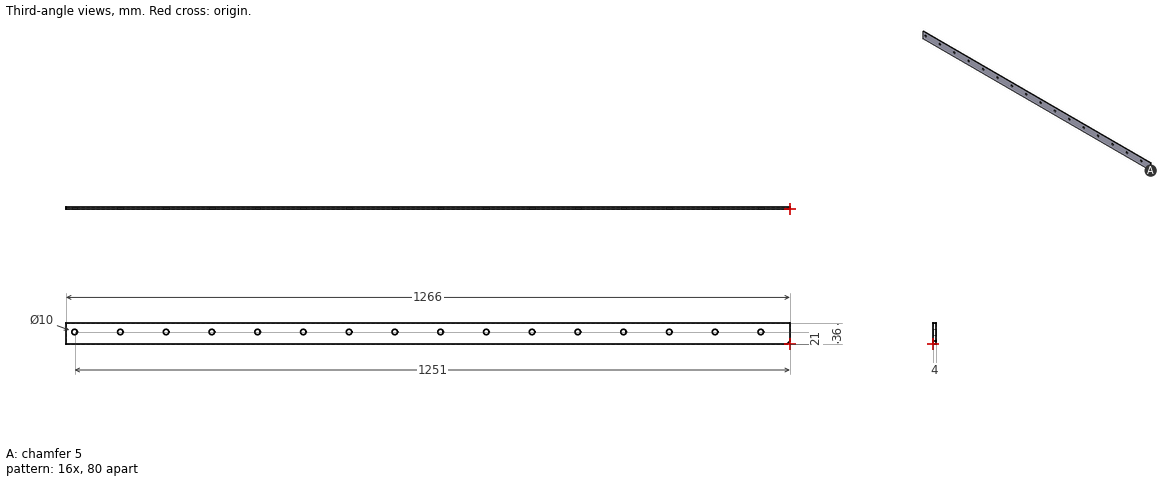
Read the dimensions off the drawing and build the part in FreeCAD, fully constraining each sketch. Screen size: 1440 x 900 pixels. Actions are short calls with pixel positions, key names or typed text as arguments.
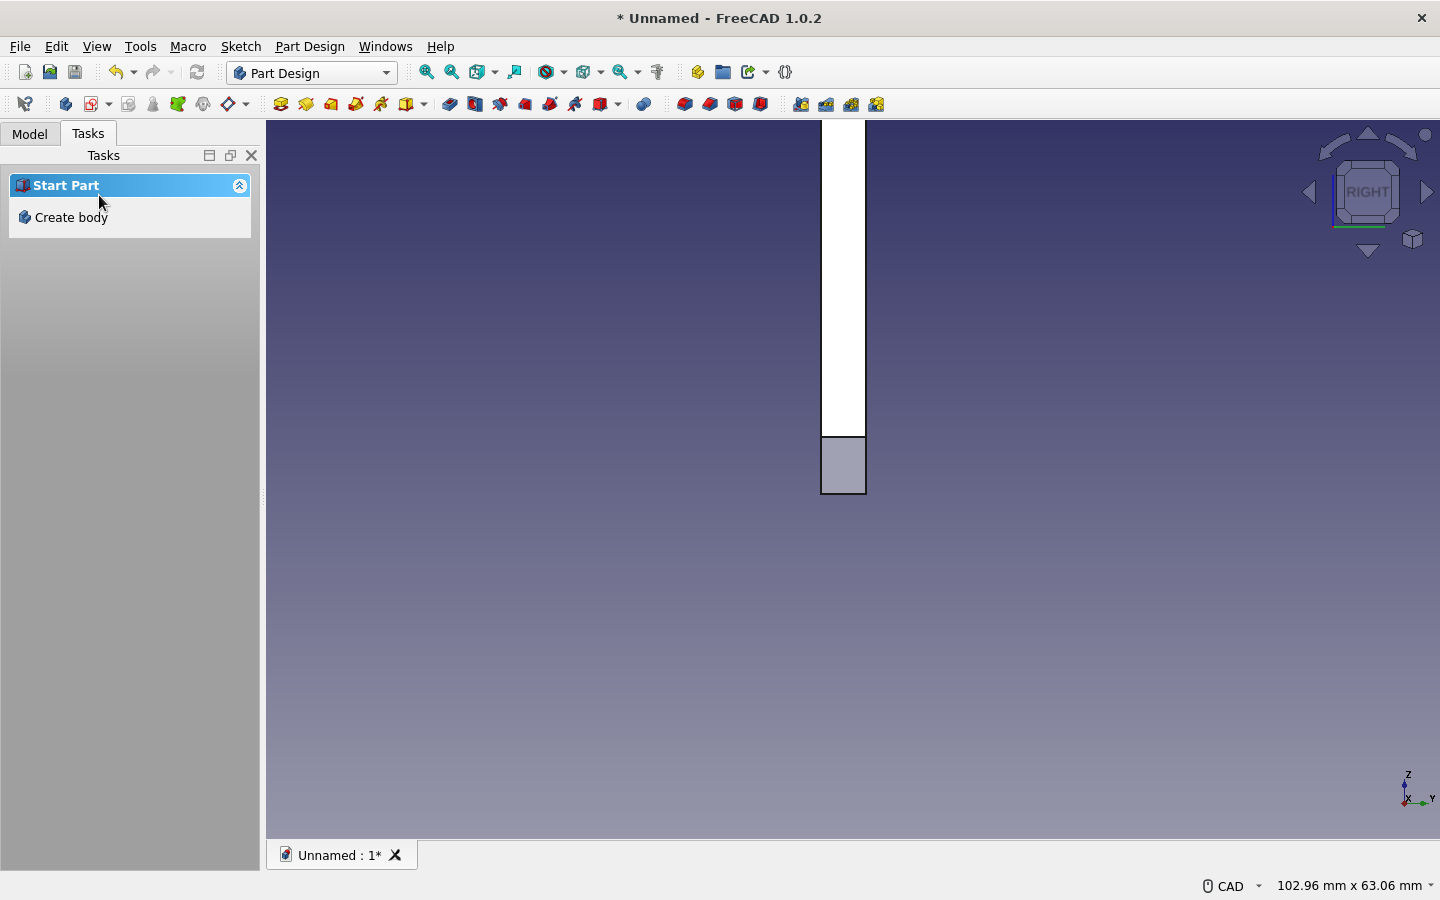
click(427, 72)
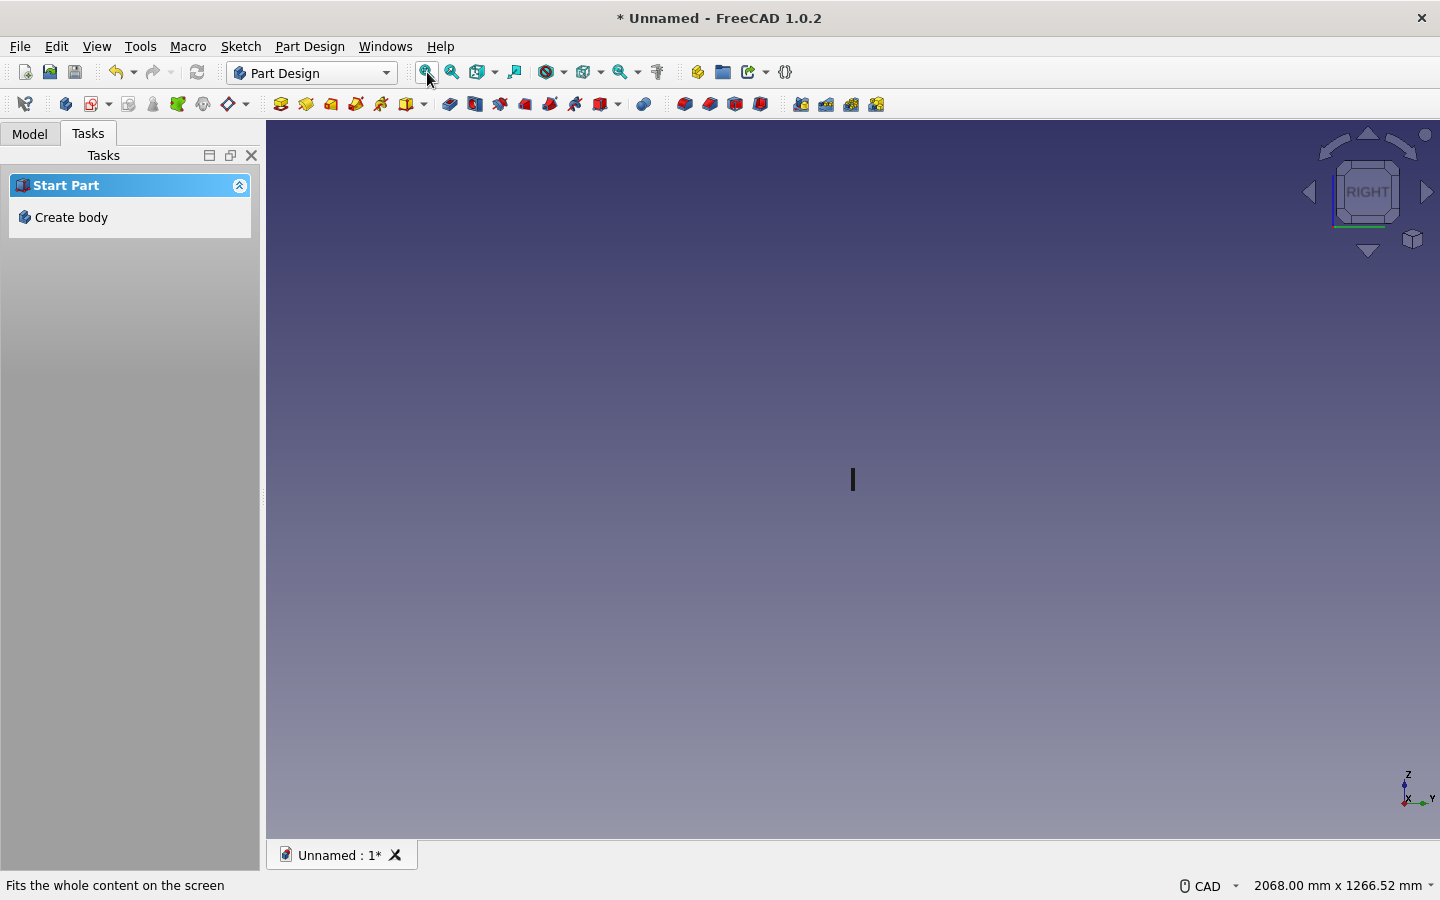
key(4)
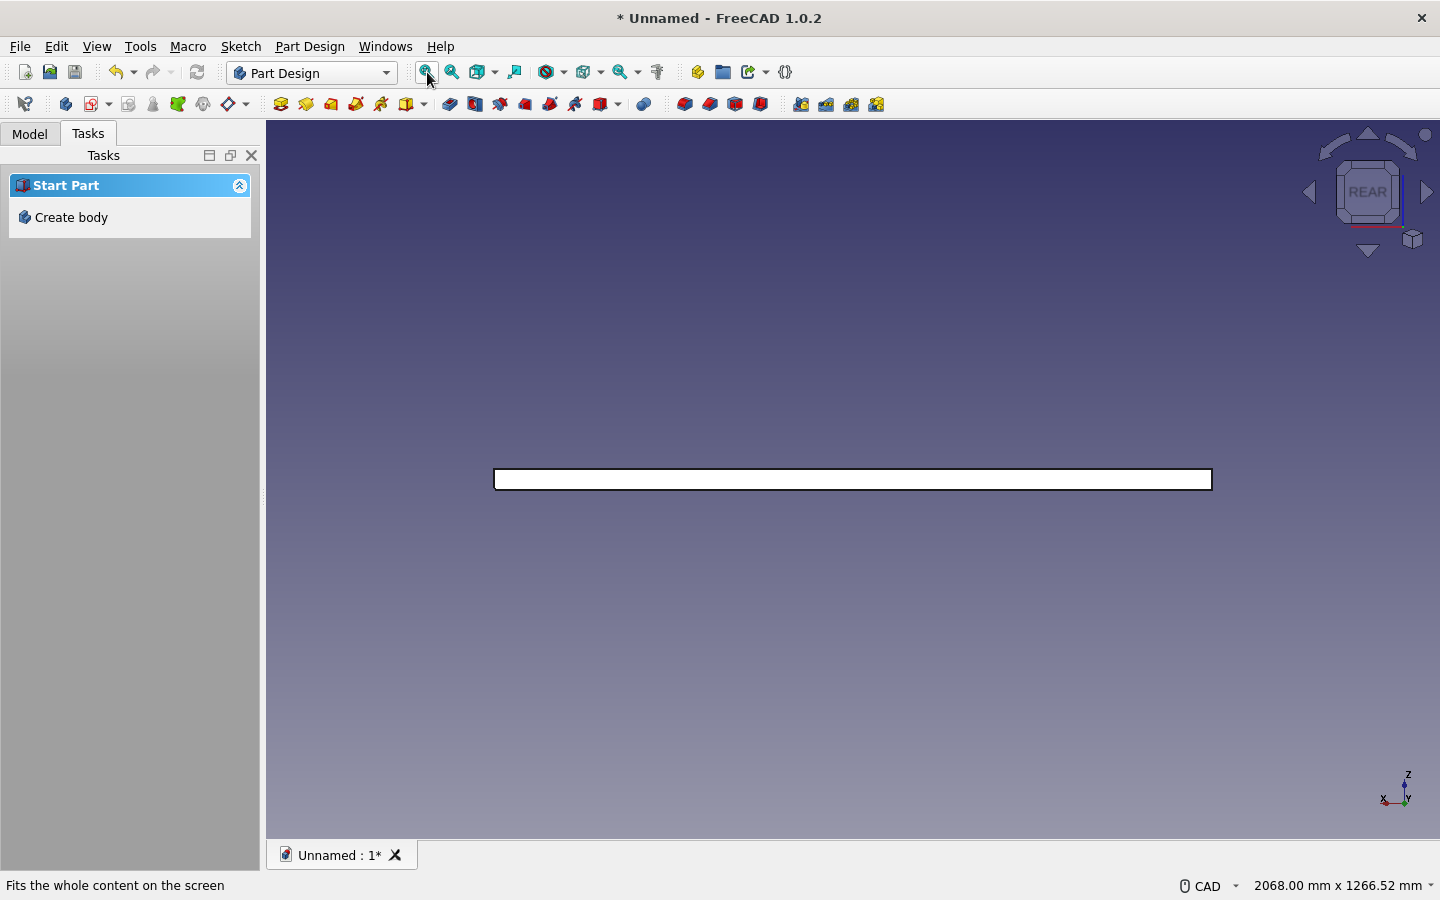
click(545, 479)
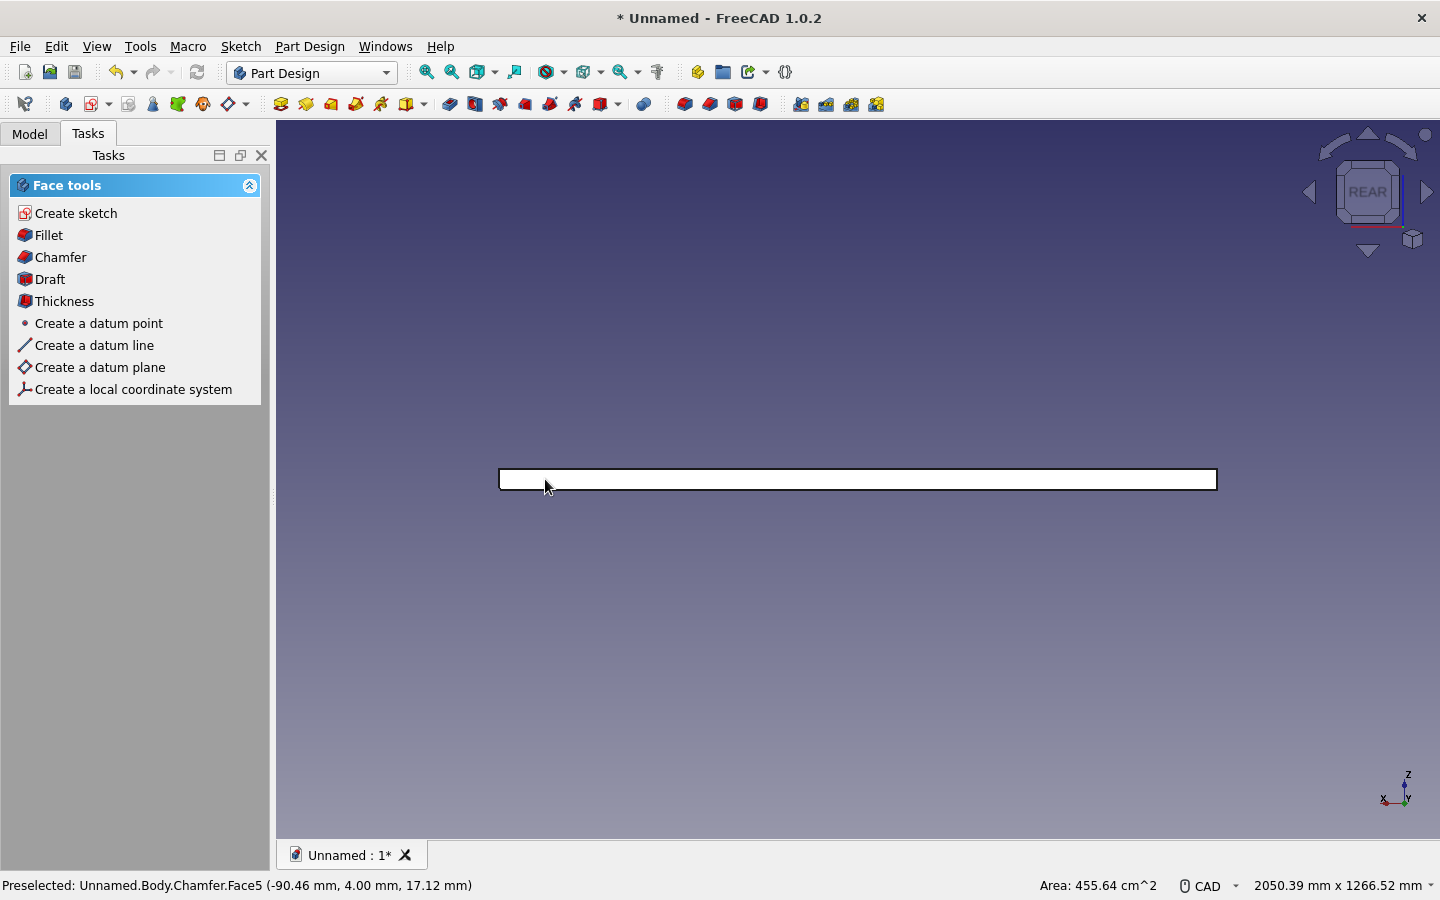
click(90, 104)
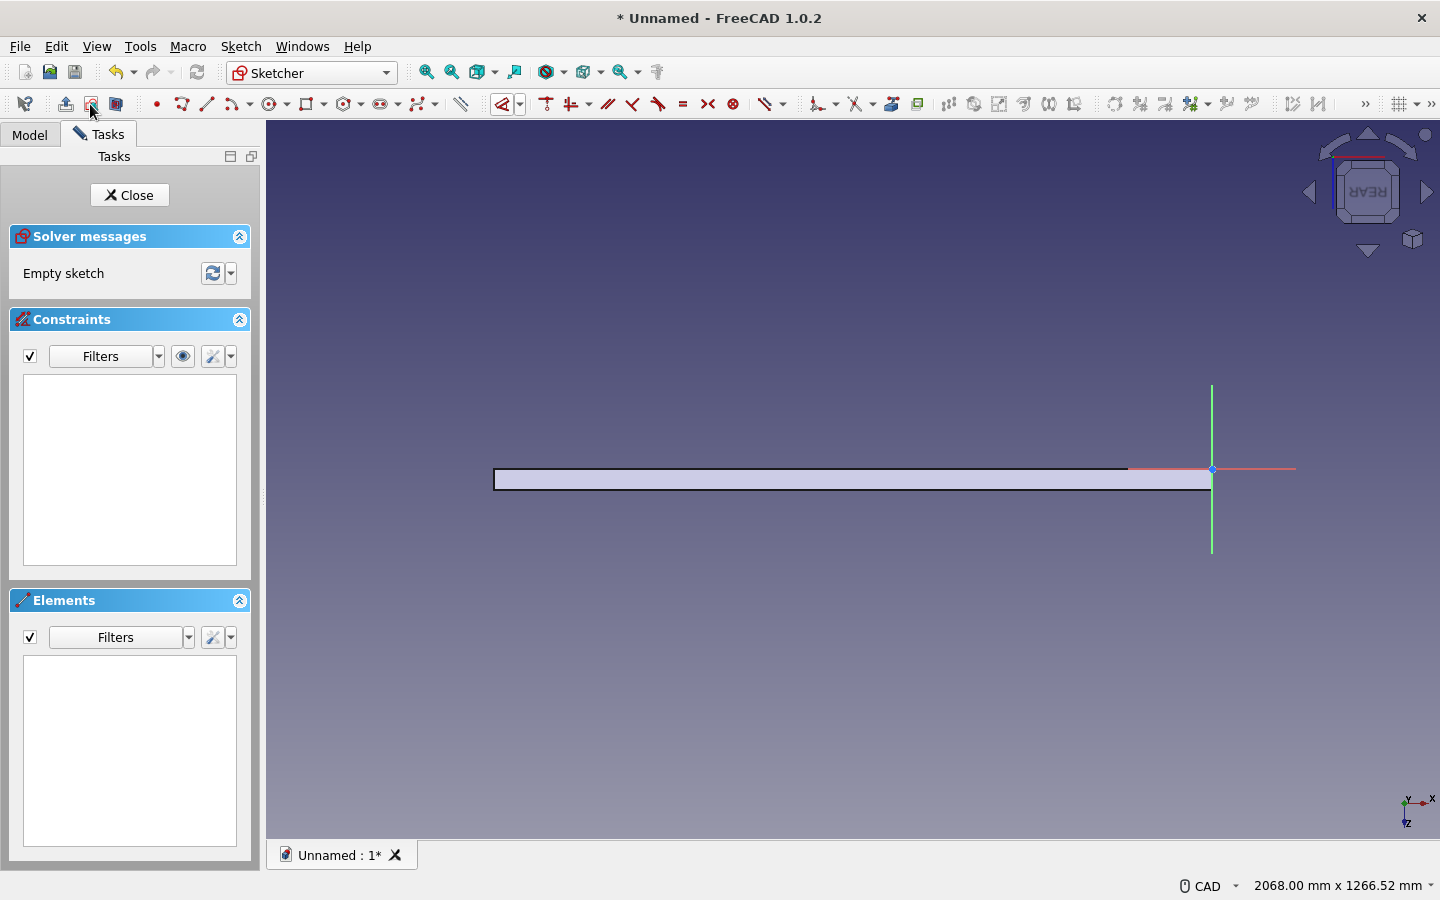
scroll(487, 481, up, 15)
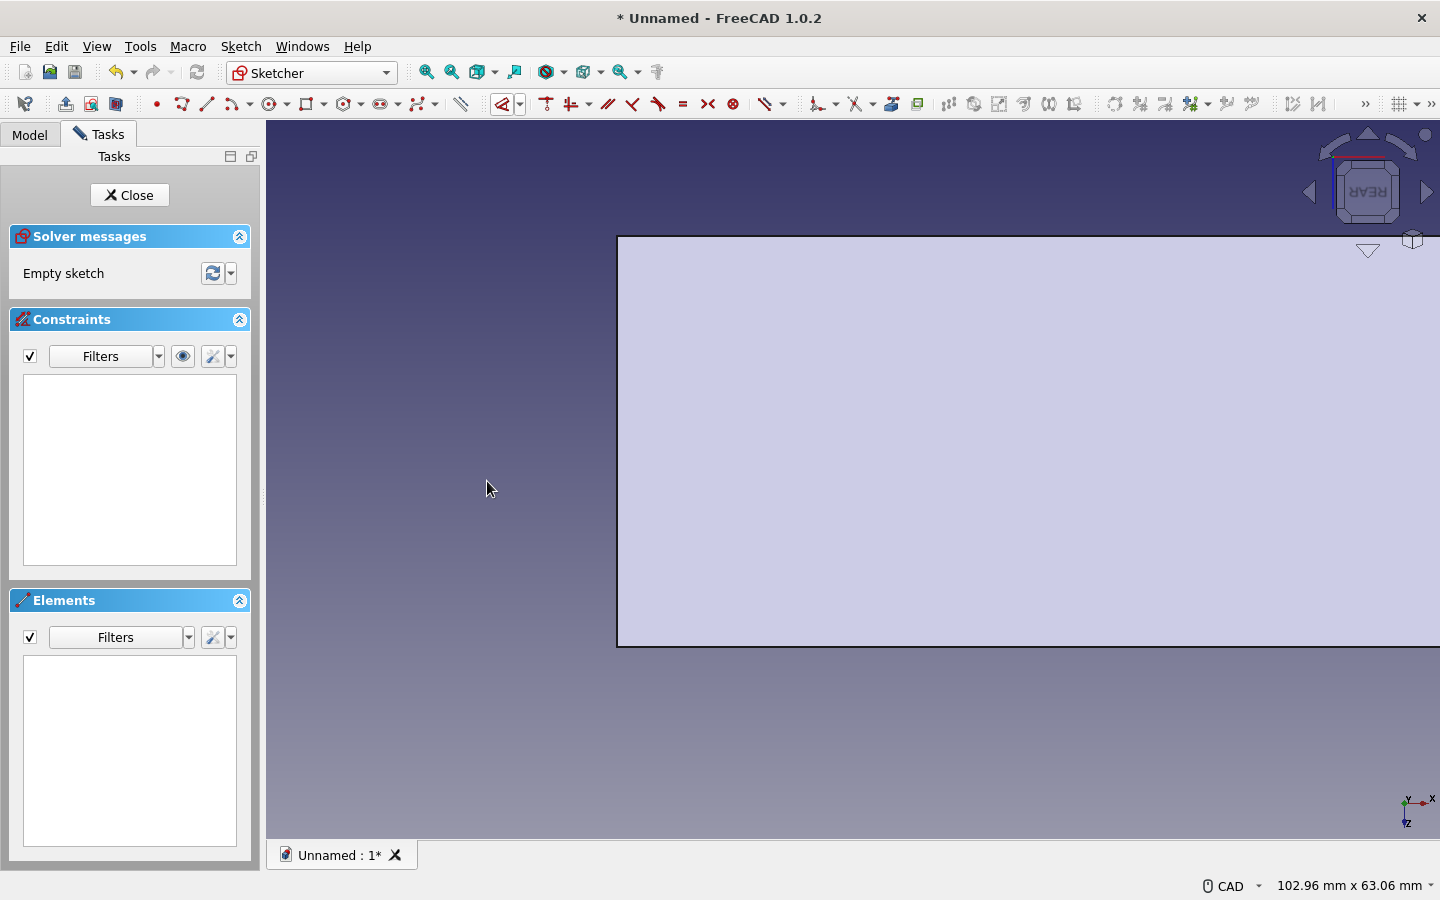
scroll(789, 474, up, 7)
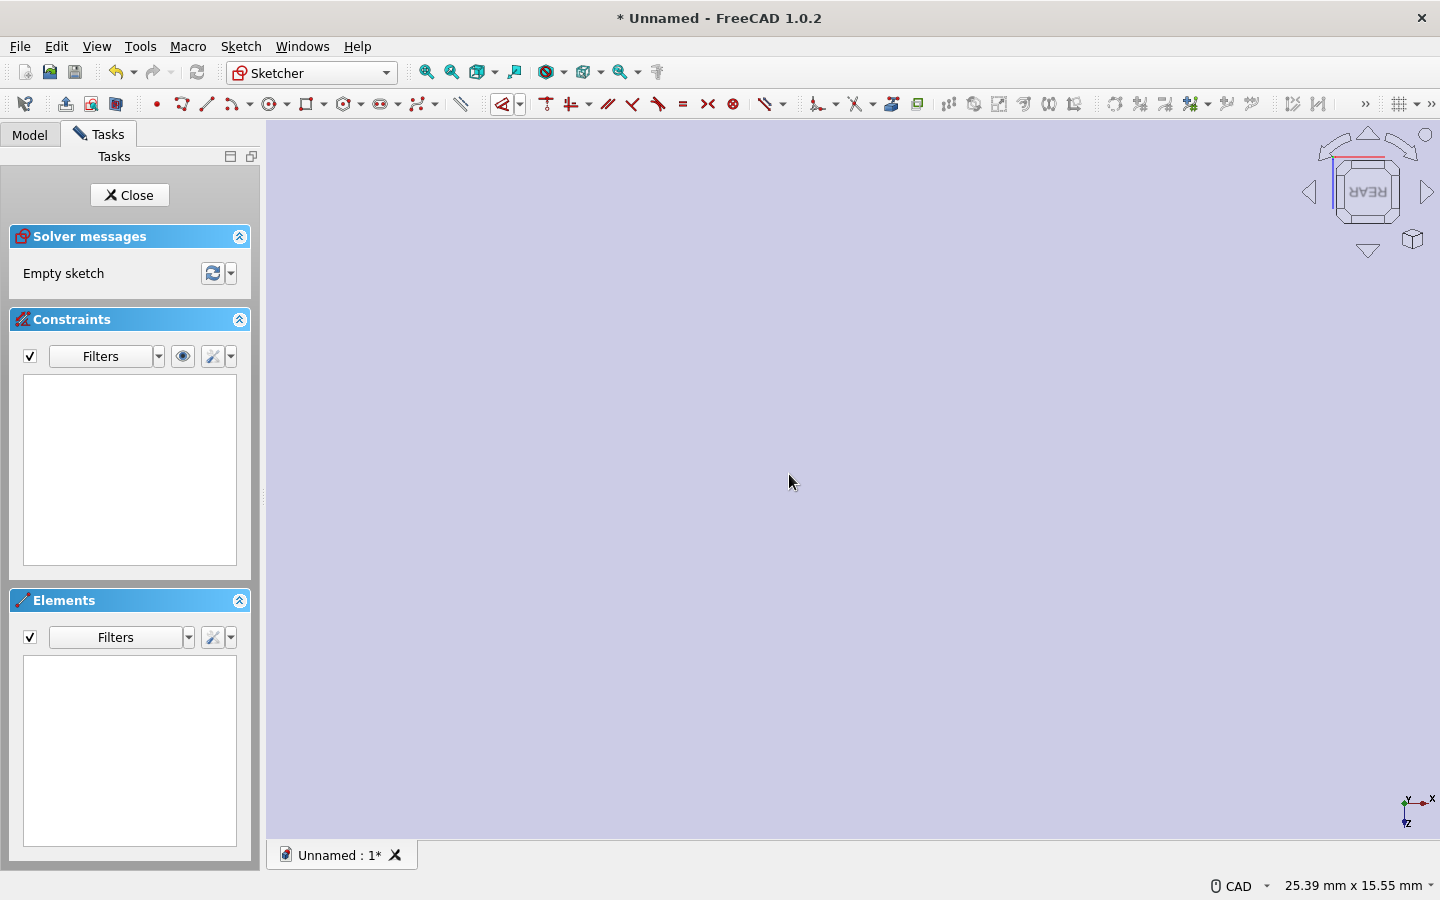
click(268, 104)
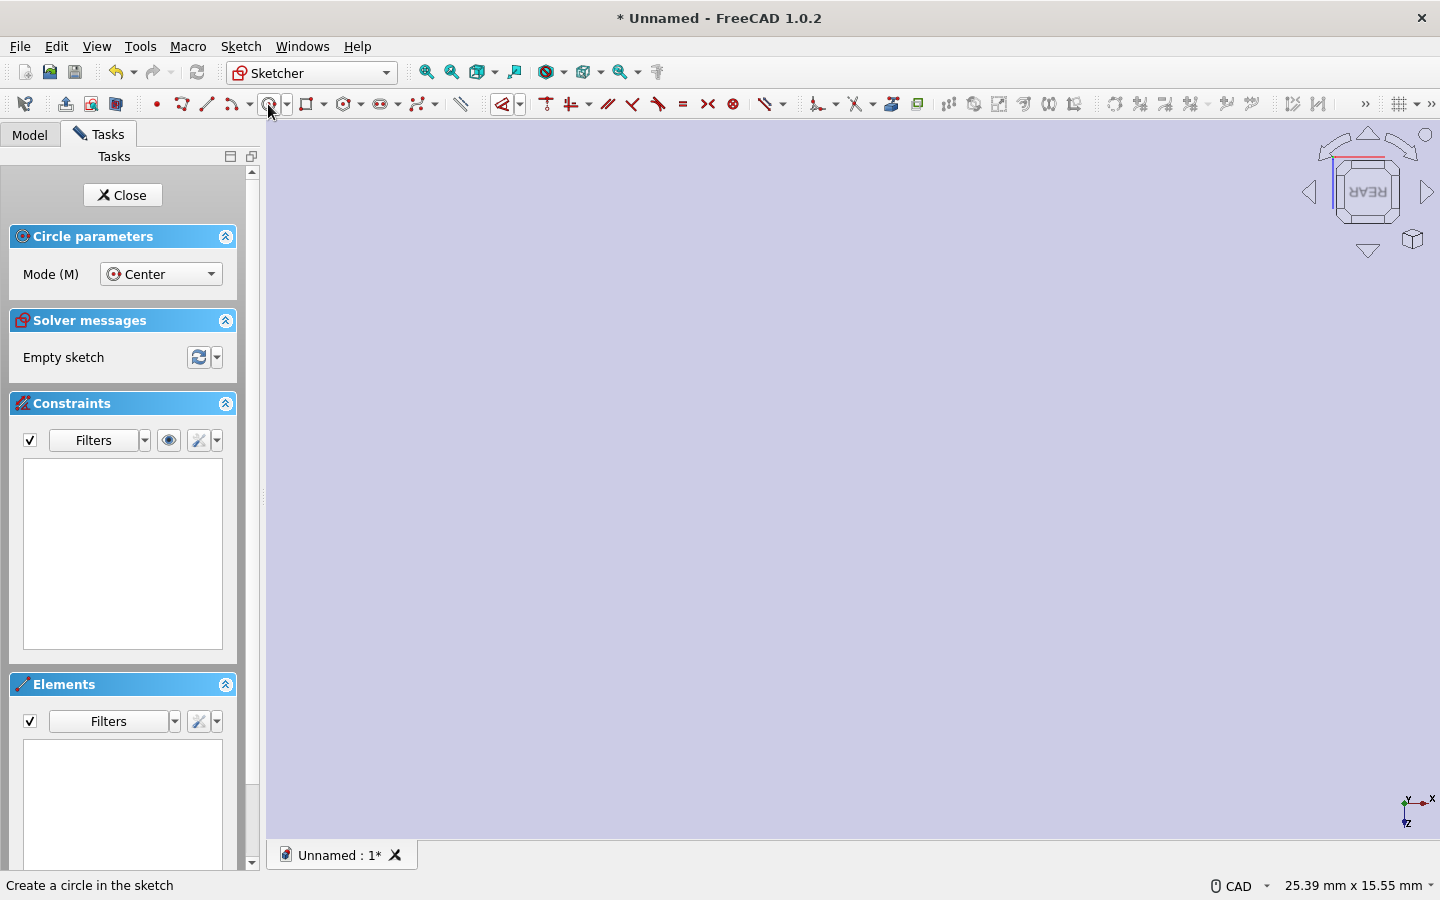
click(783, 479)
click(947, 315)
key(Escape)